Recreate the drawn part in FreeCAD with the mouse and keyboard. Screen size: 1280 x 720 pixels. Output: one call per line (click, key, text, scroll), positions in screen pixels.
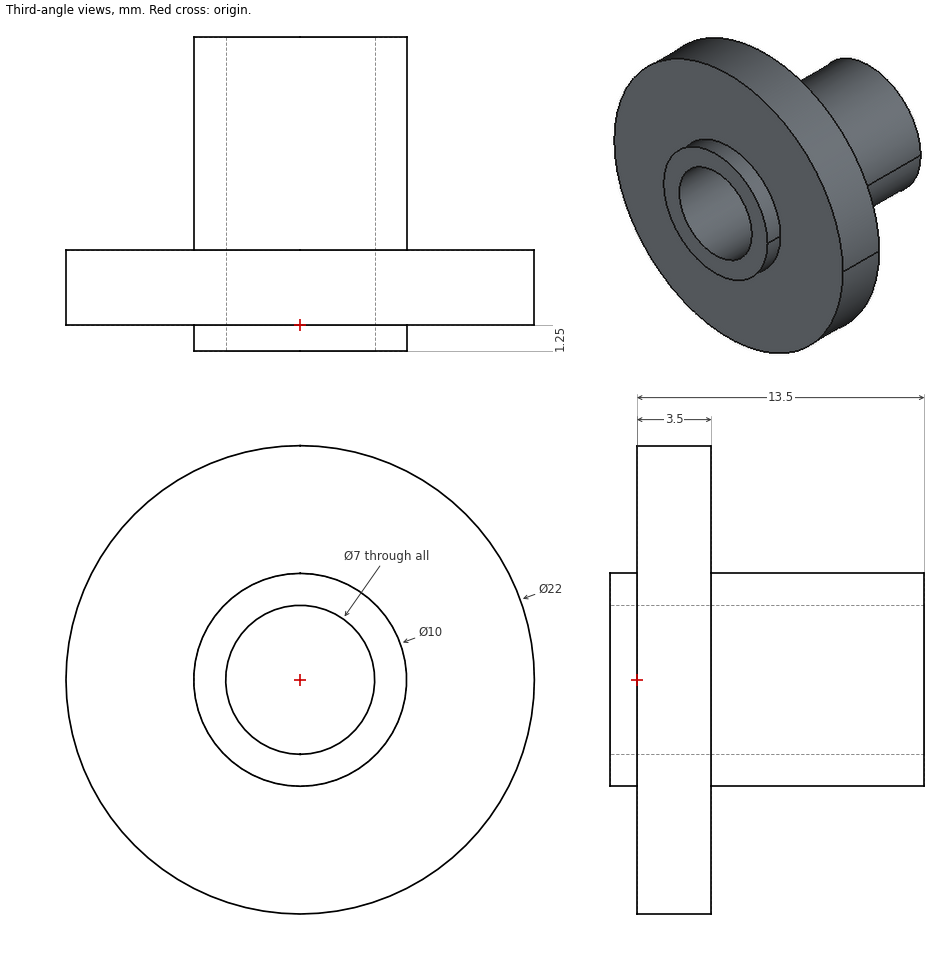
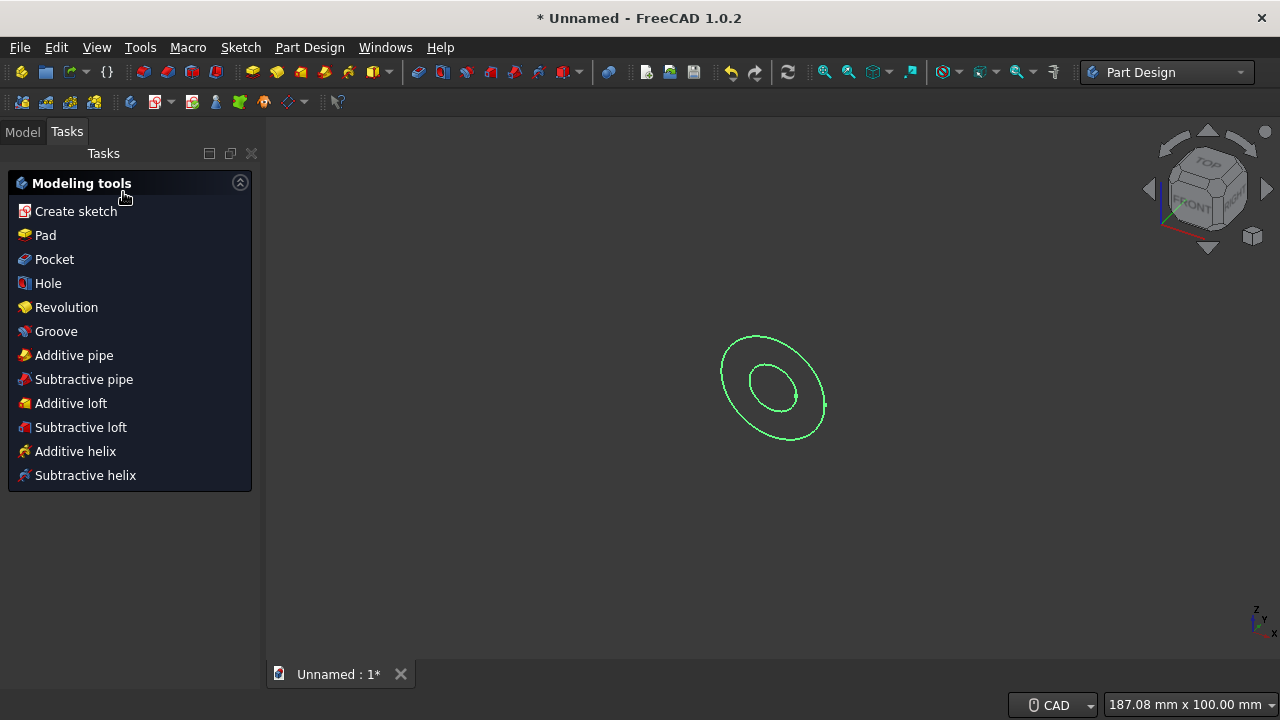
click(254, 72)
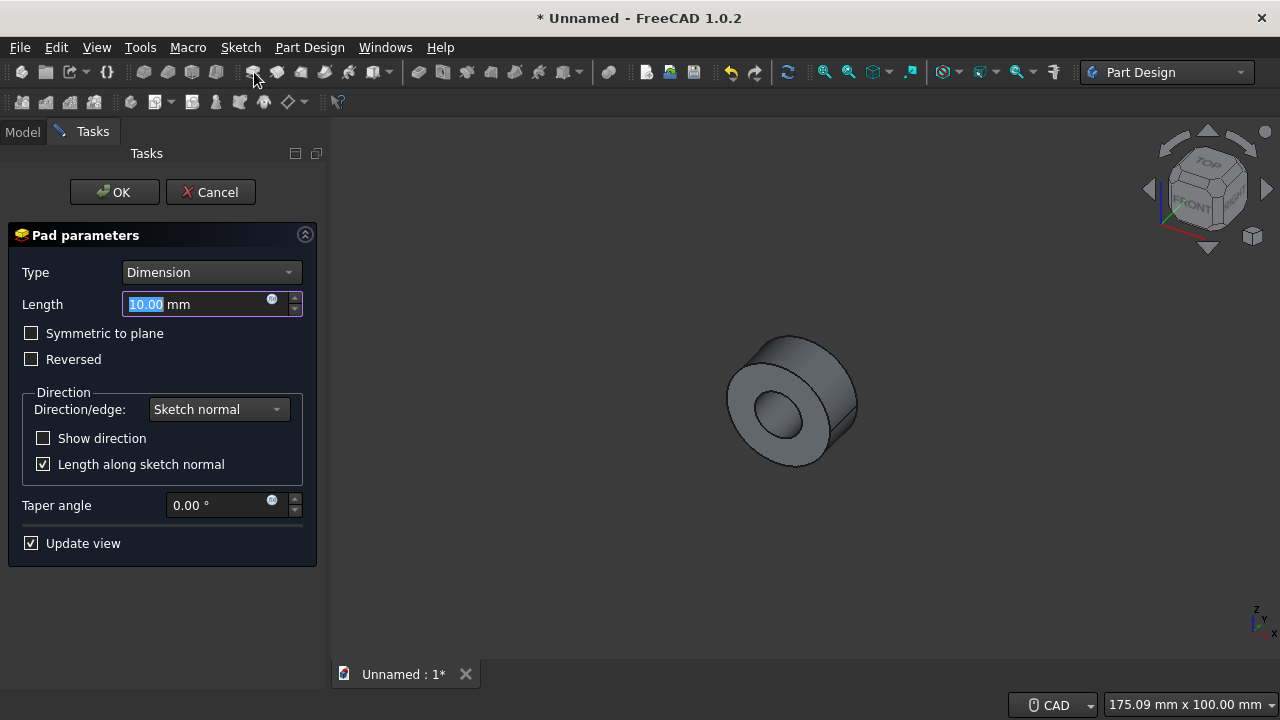
text(3.5)
key(Tab)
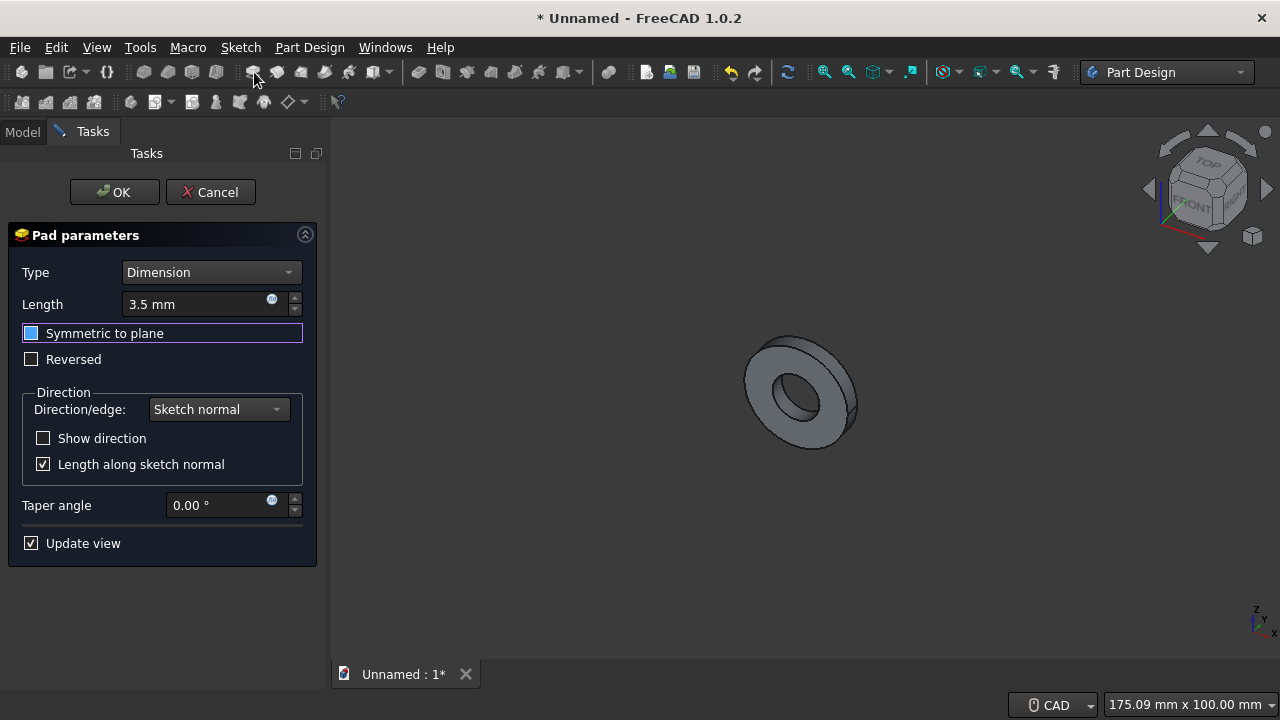
click(30, 359)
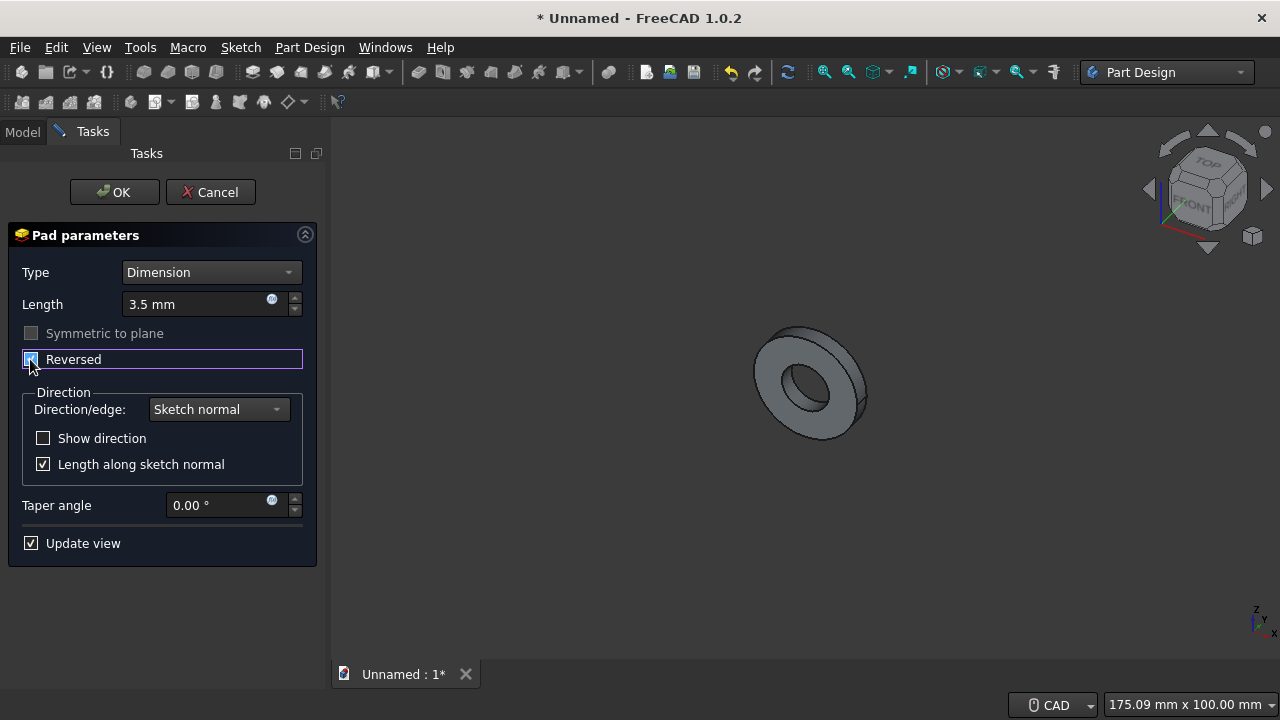
click(115, 192)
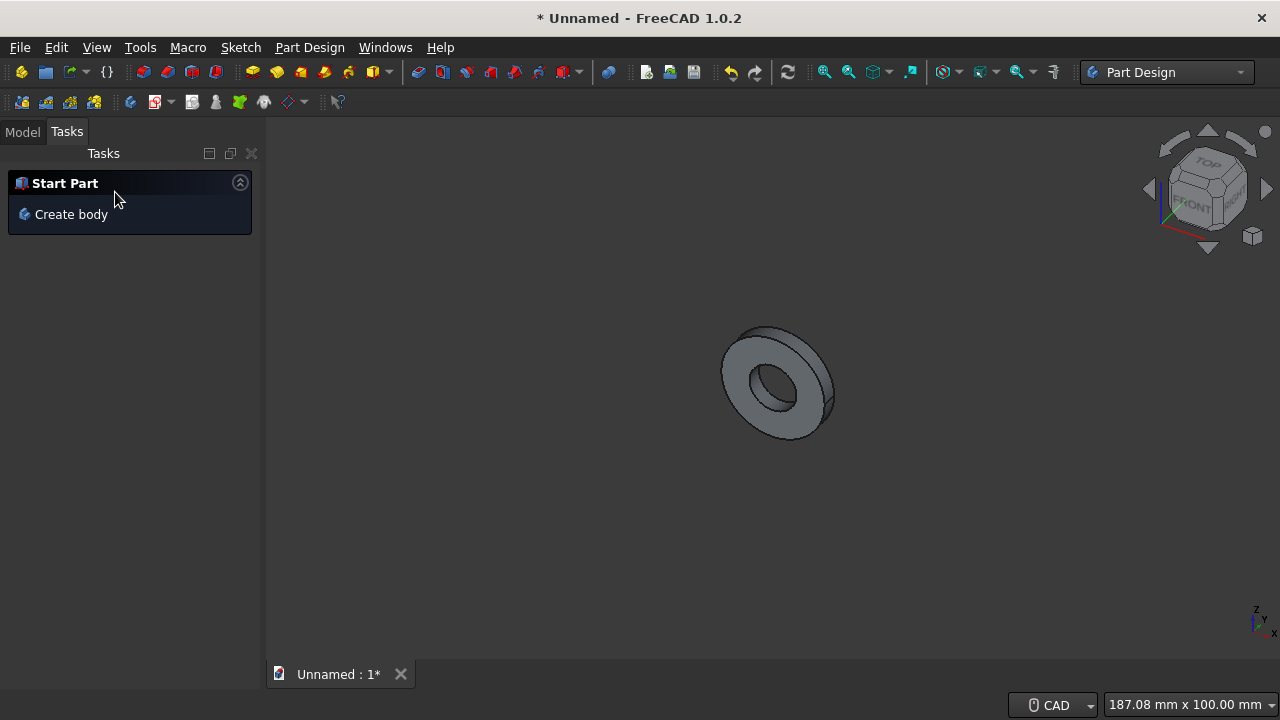
key(v)
key(f)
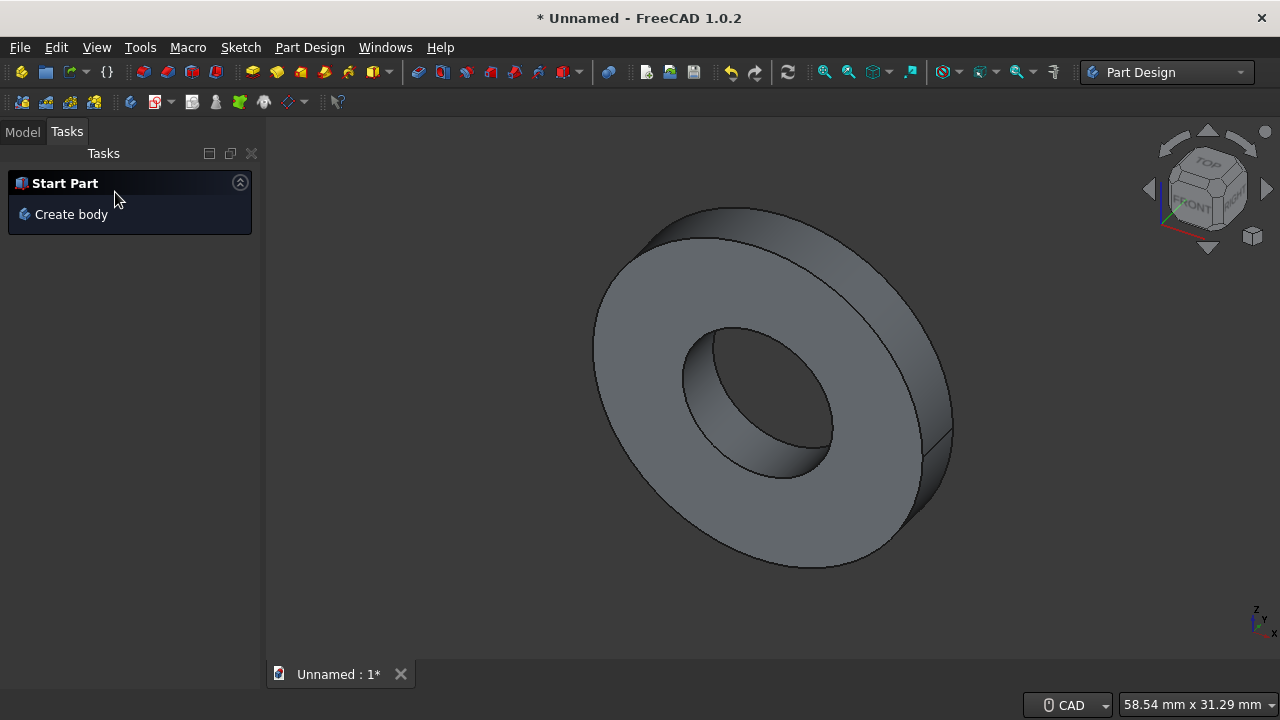
click(132, 102)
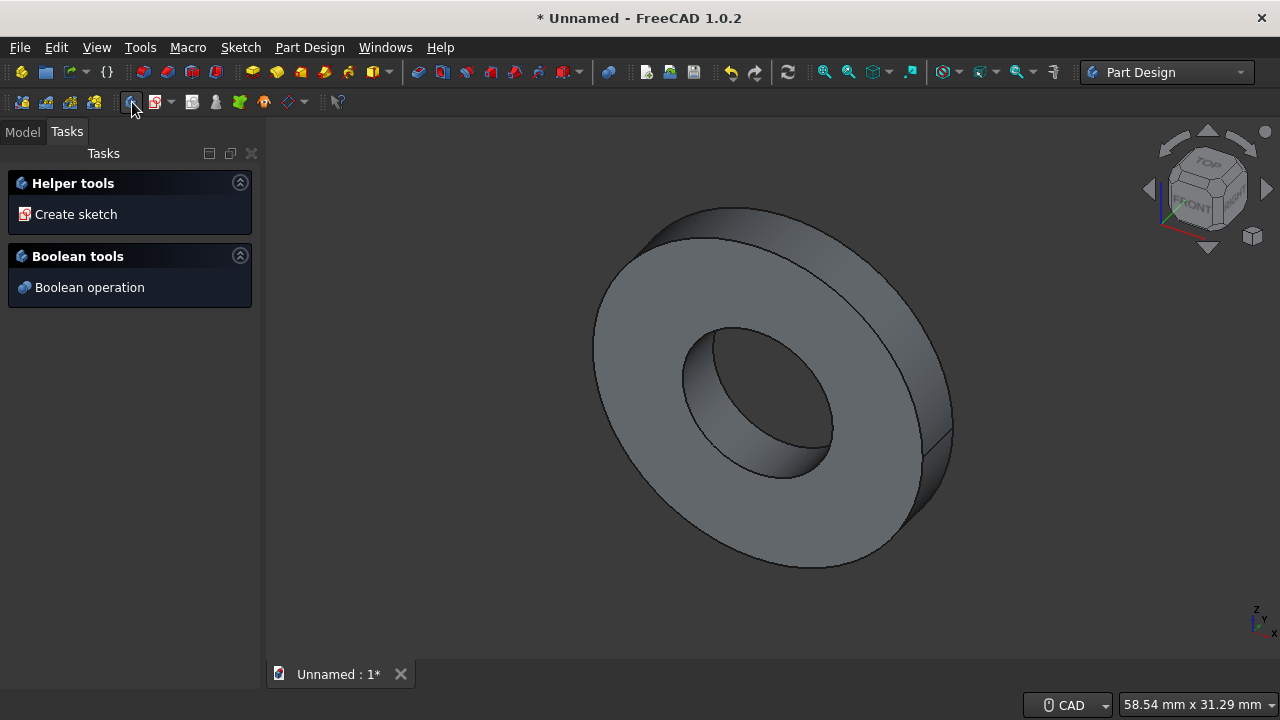
click(306, 619)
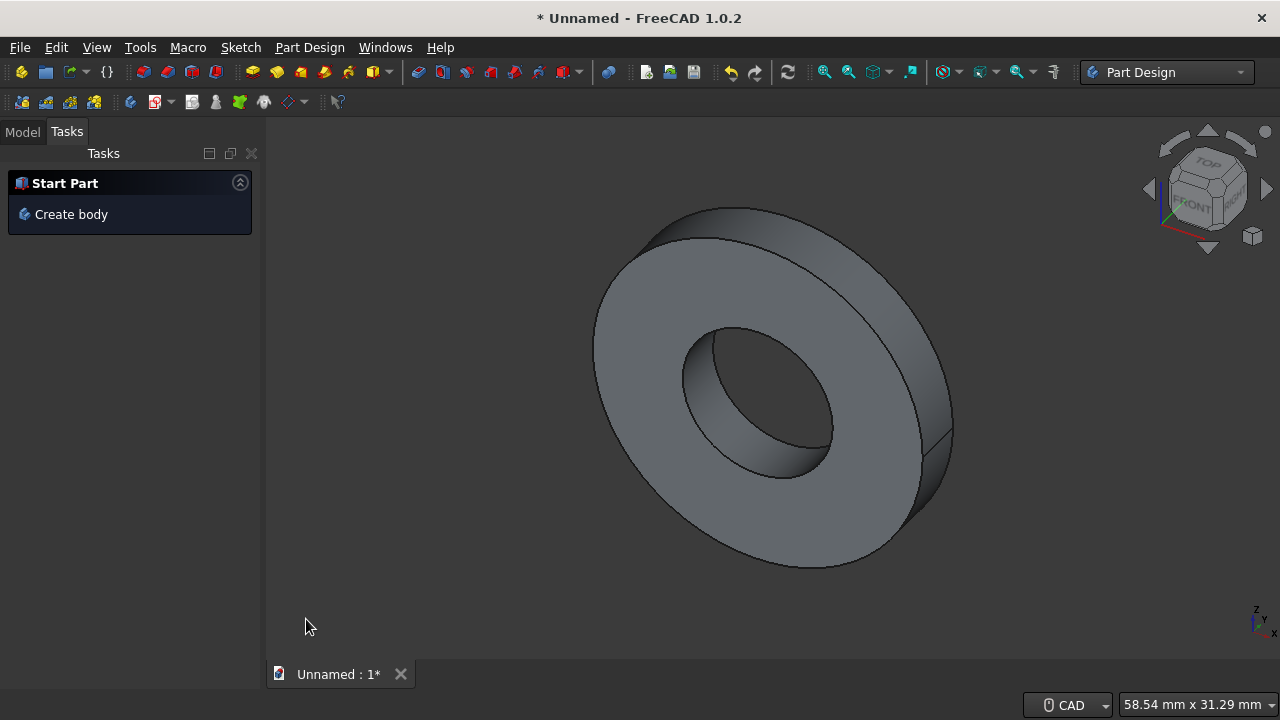
click(156, 102)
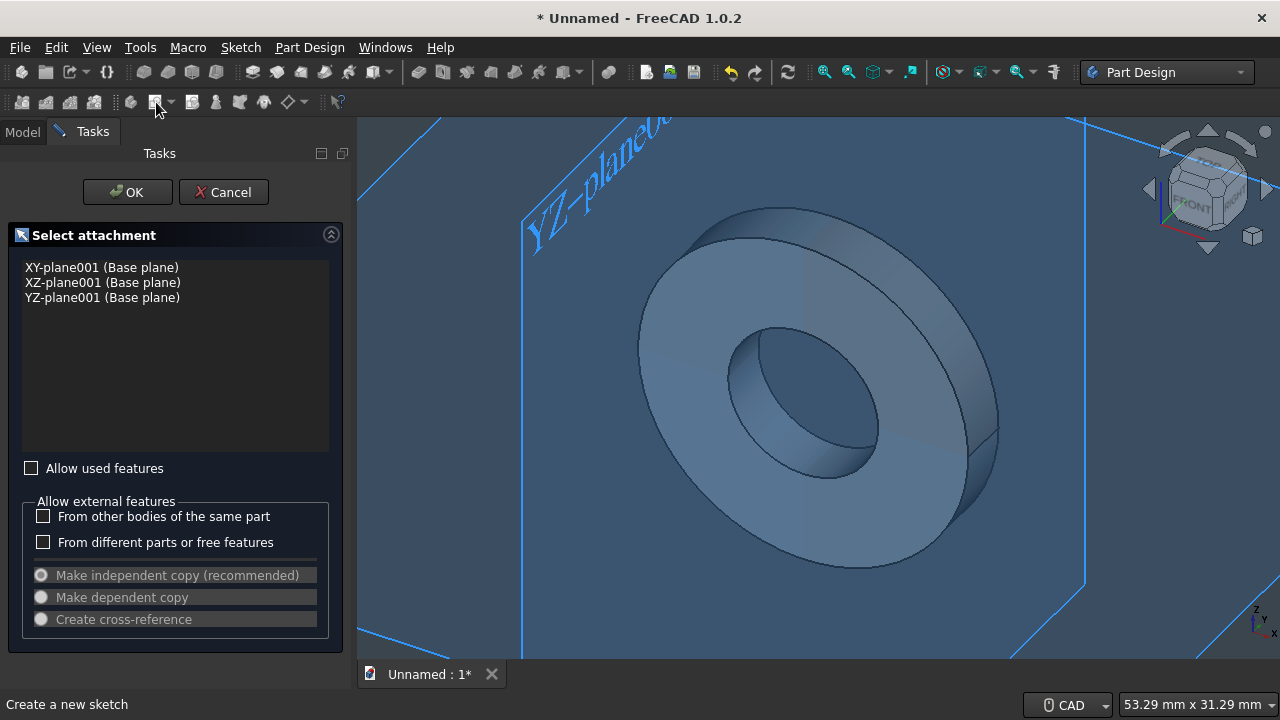
click(82, 282)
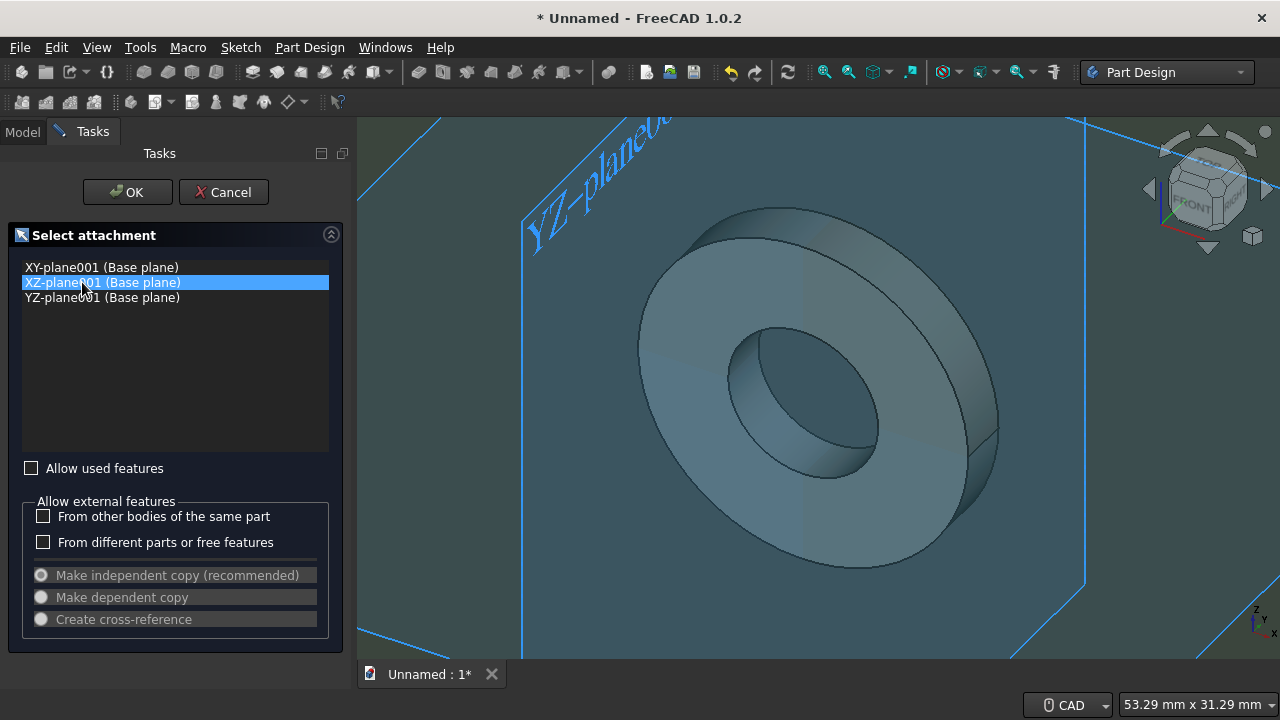
click(128, 192)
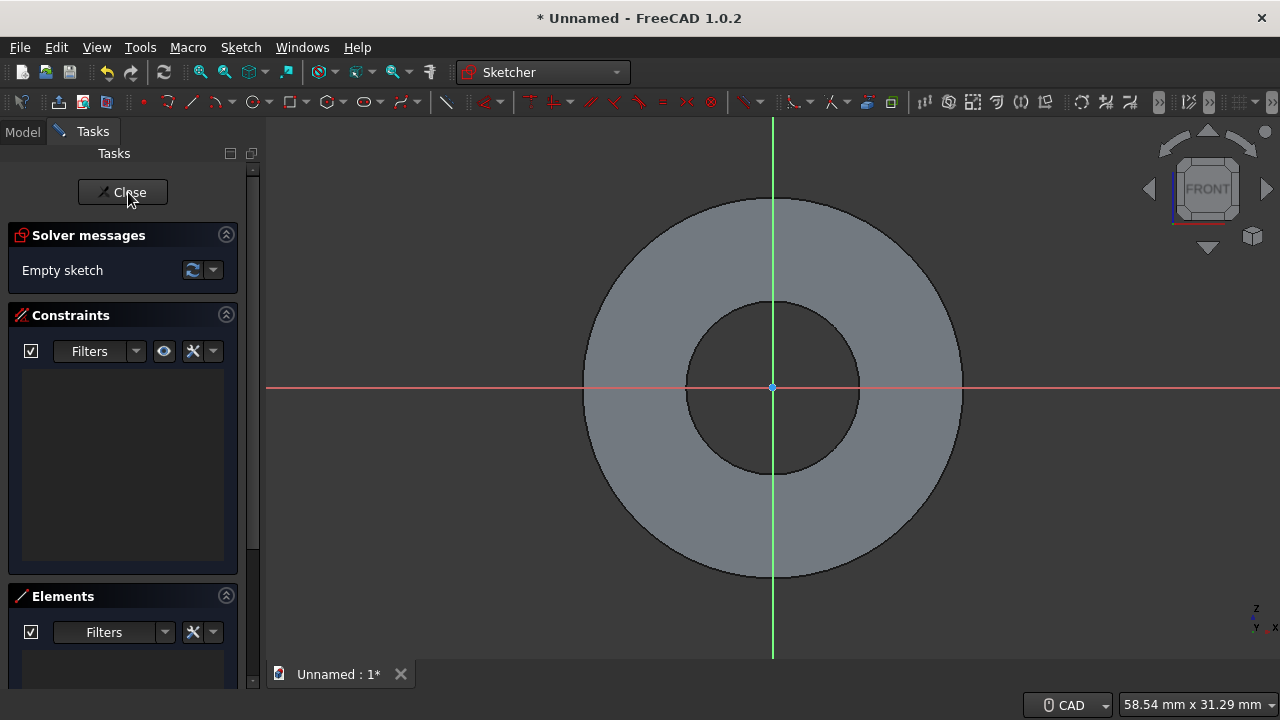
scroll(856, 388, up, 3)